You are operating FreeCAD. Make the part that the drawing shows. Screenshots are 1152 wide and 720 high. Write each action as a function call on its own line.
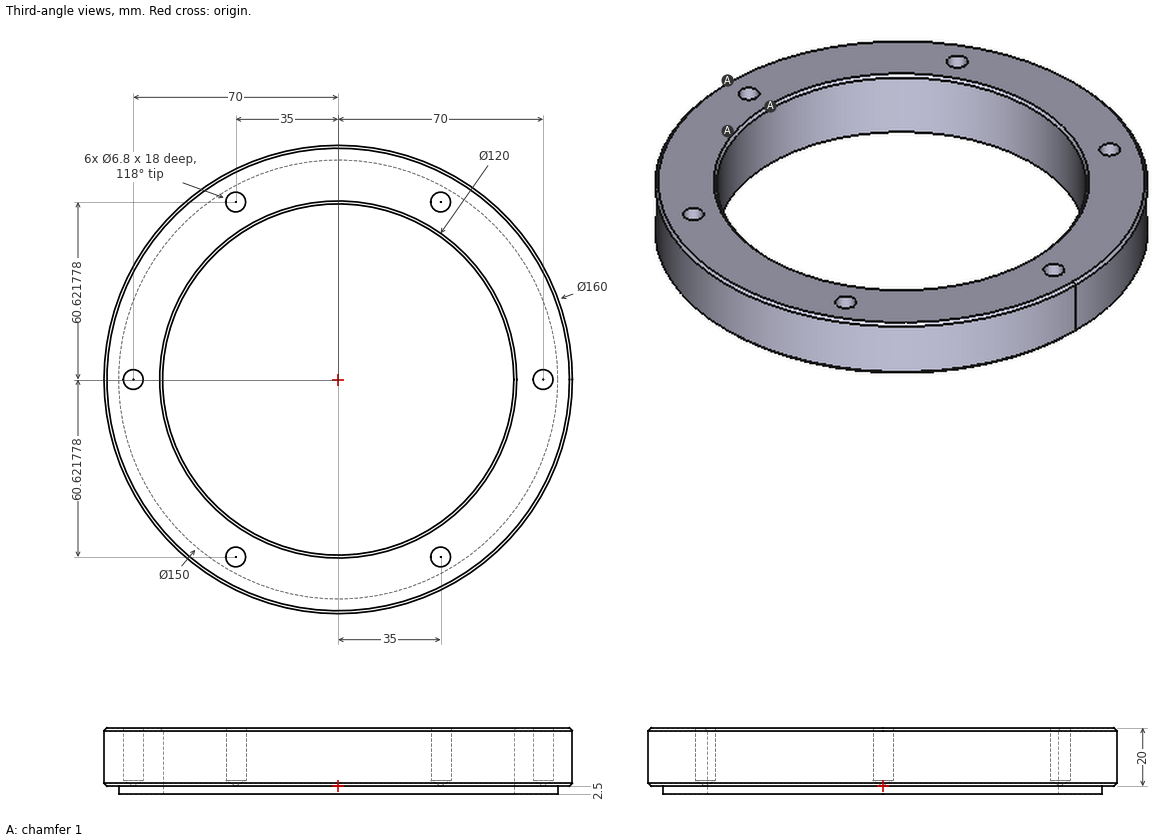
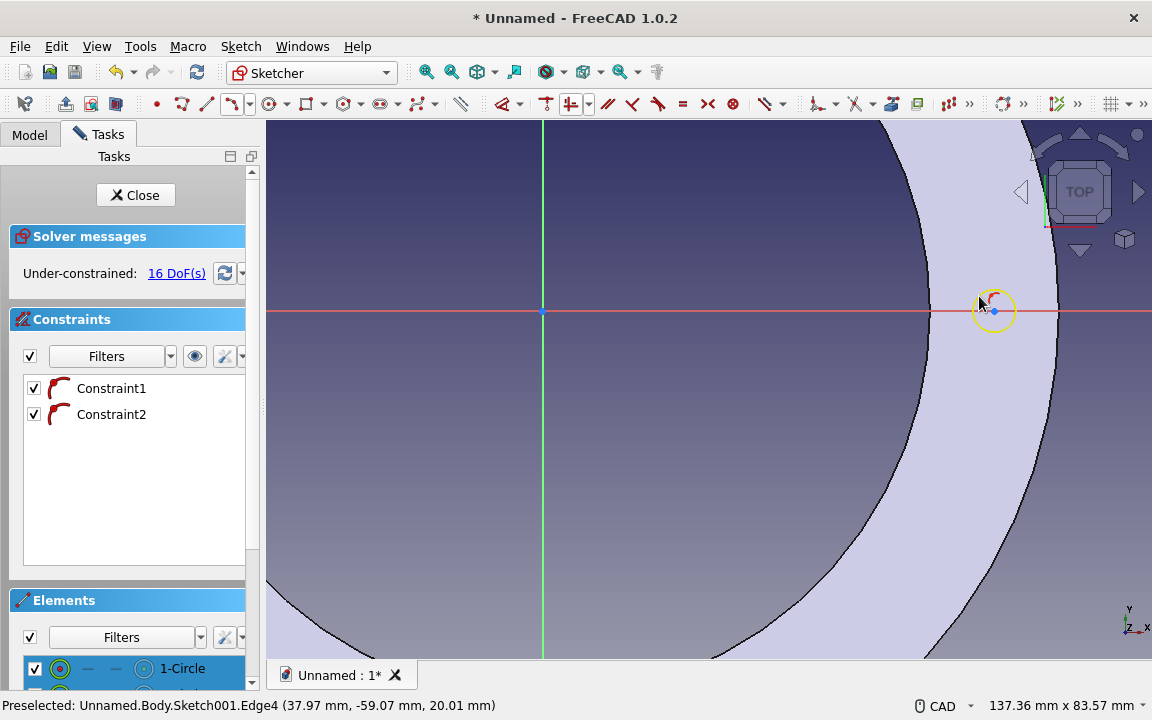
click(979, 296)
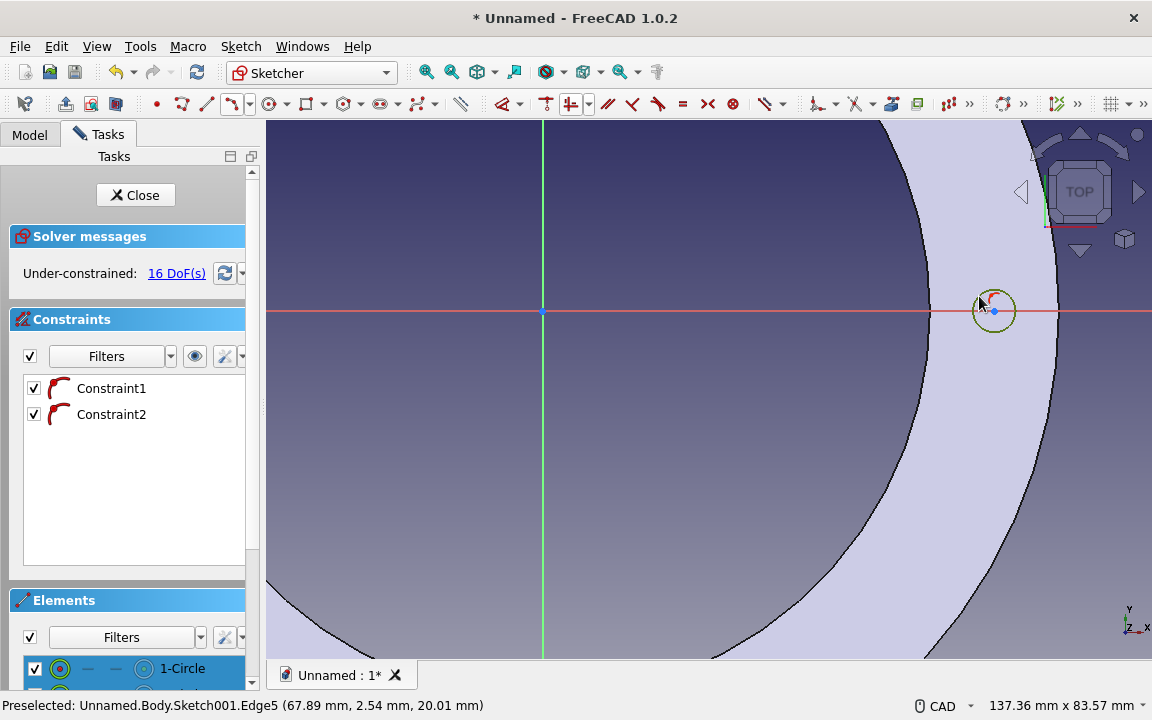
scroll(720, 454, down, 4)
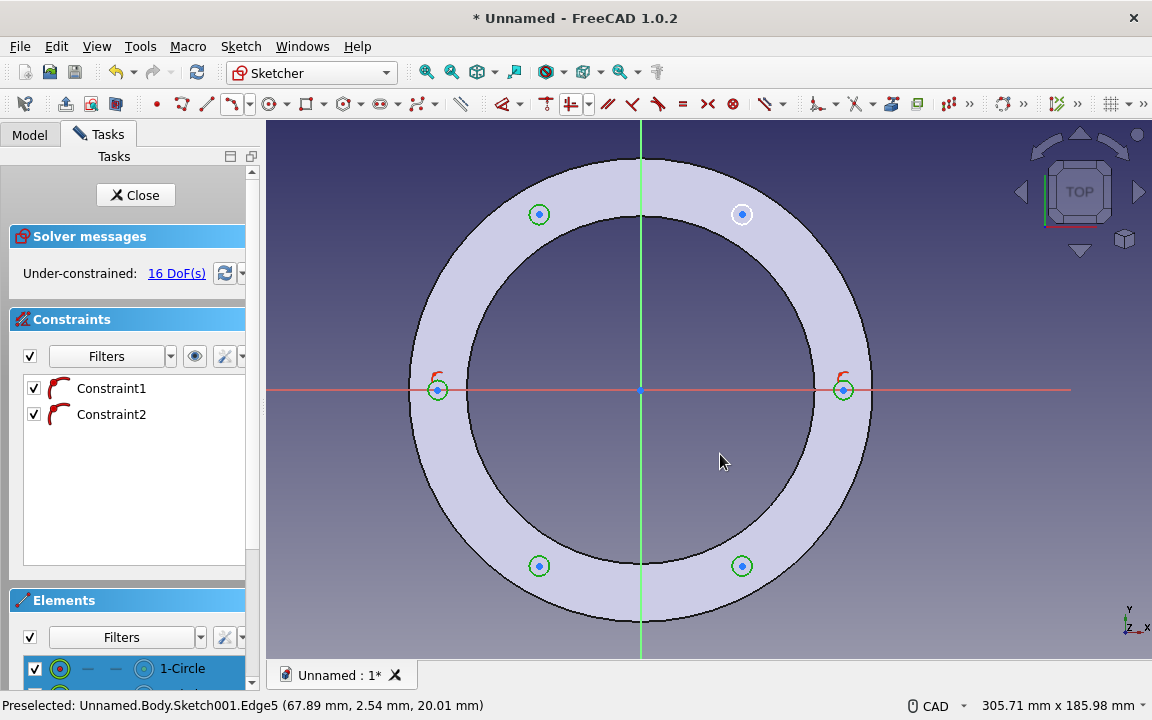
scroll(749, 208, up, 2)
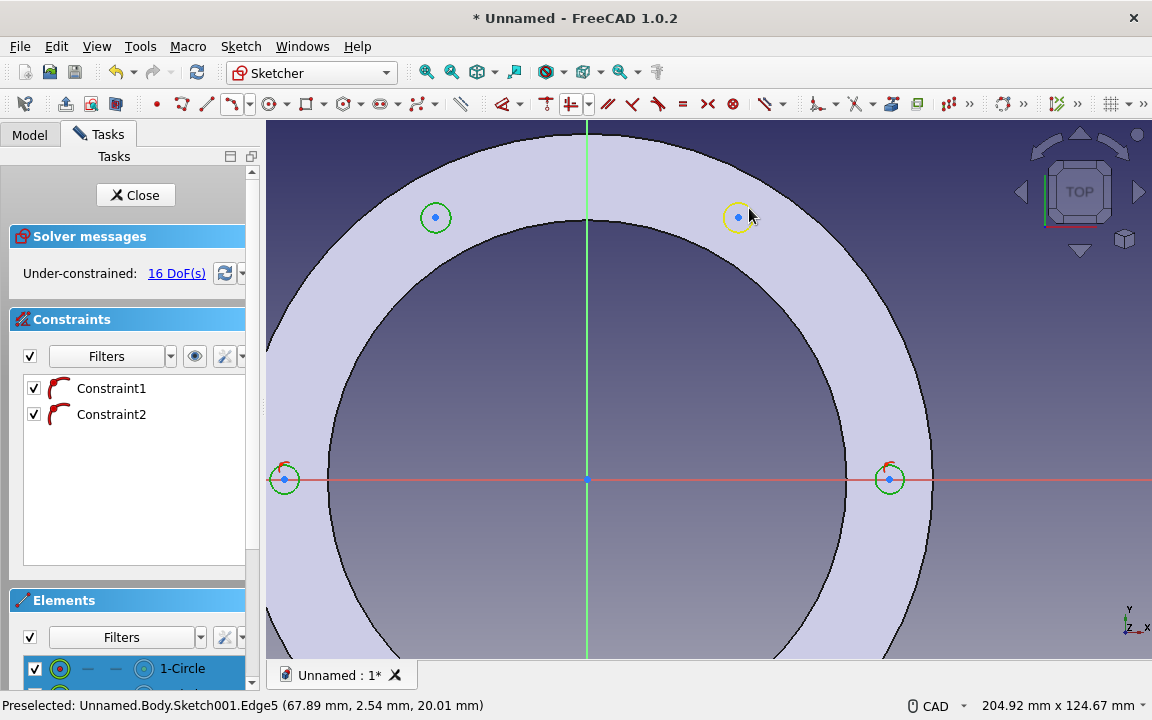
click(749, 207)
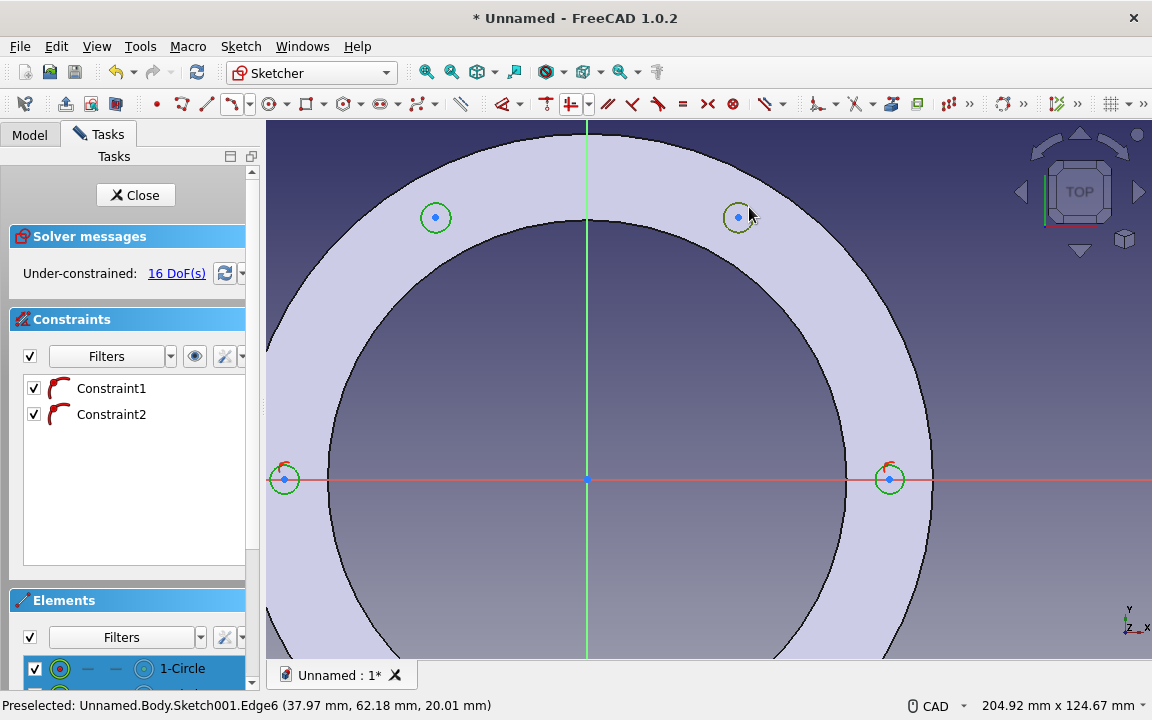
key(e)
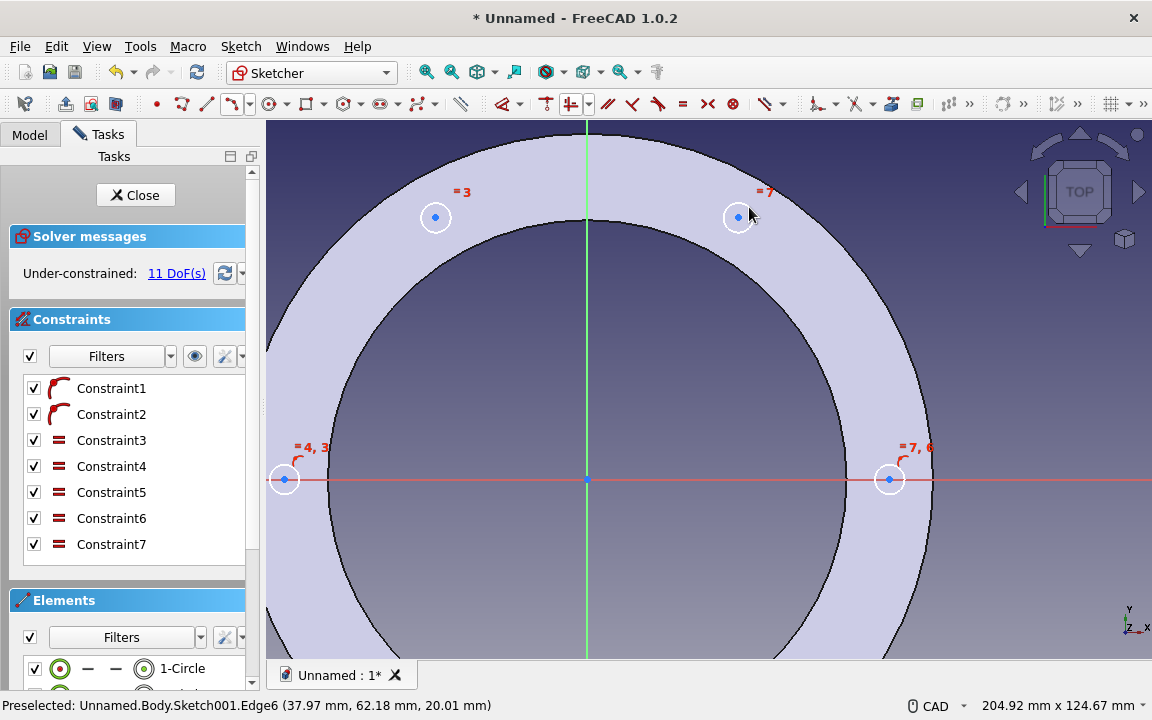
click(436, 218)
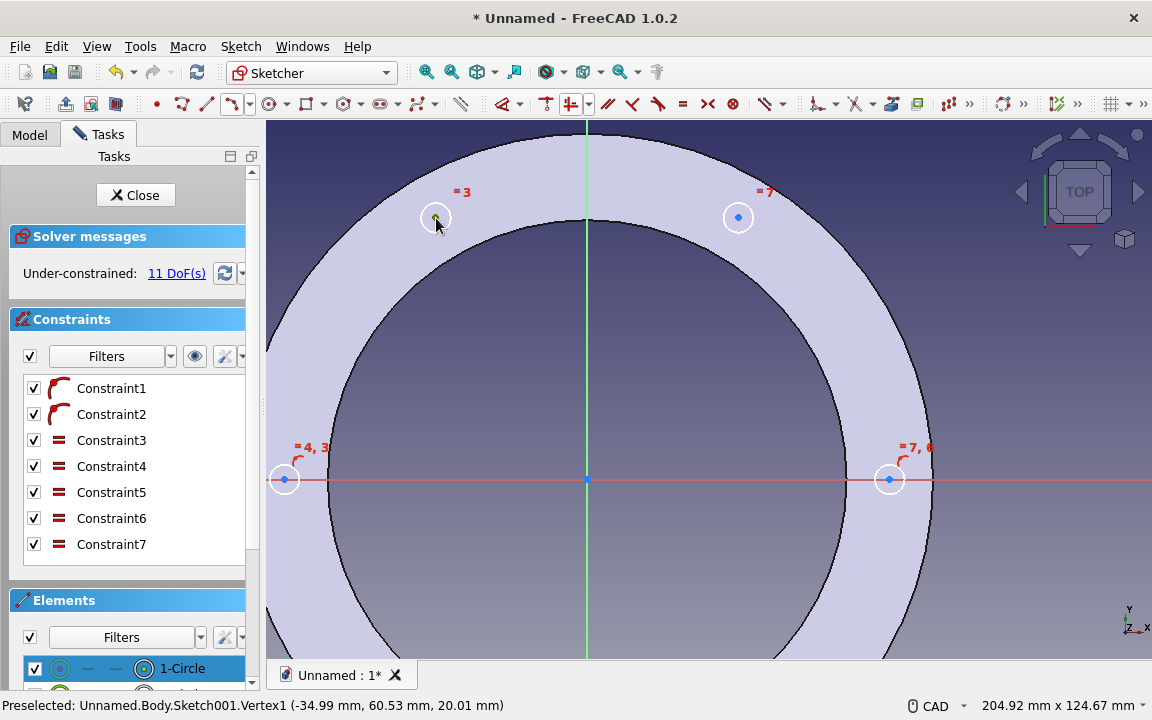
scroll(749, 206, down, 2)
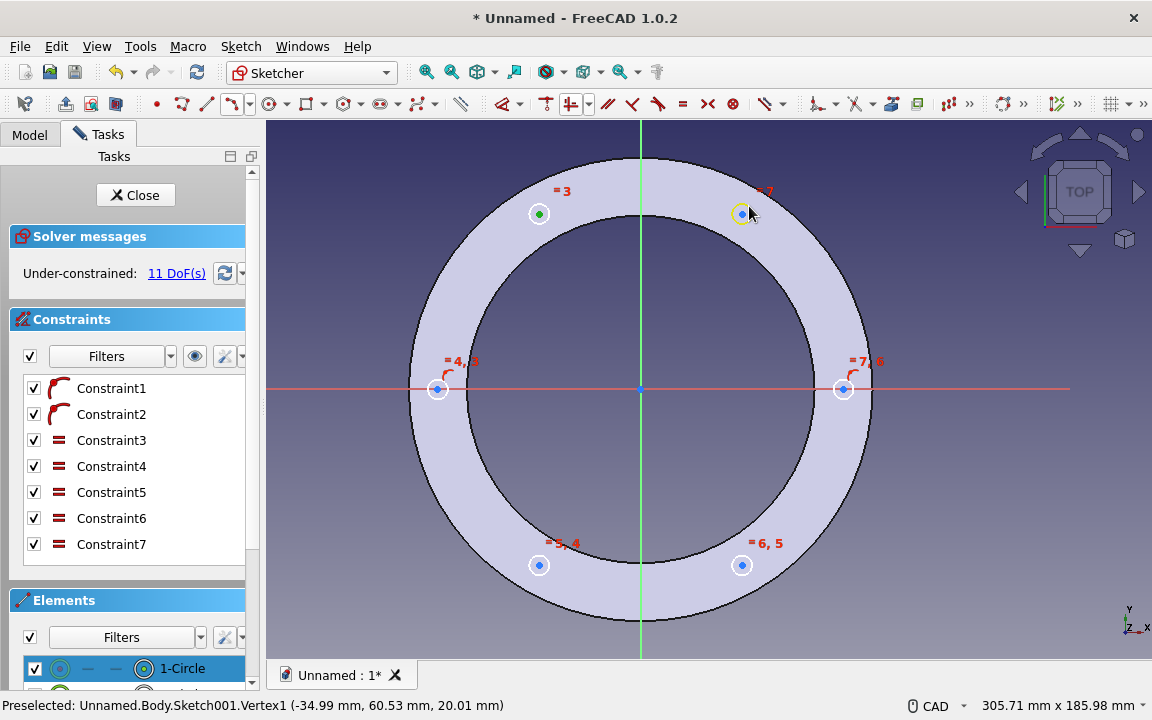
click(539, 565)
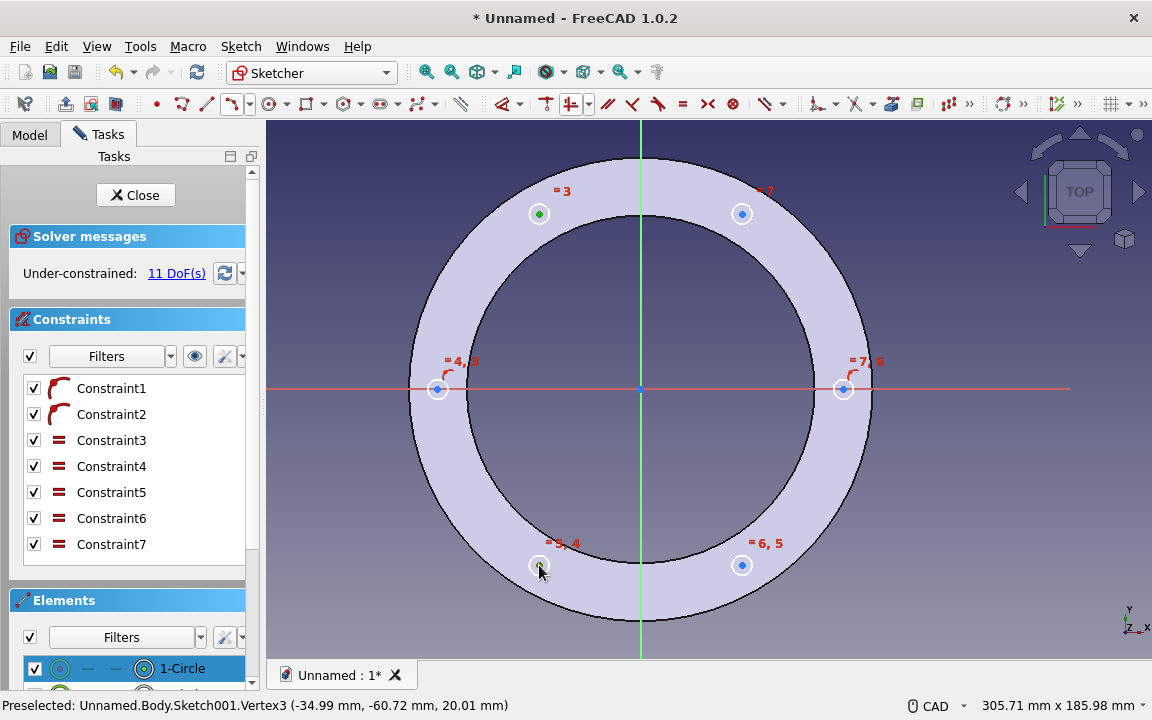
click(588, 104)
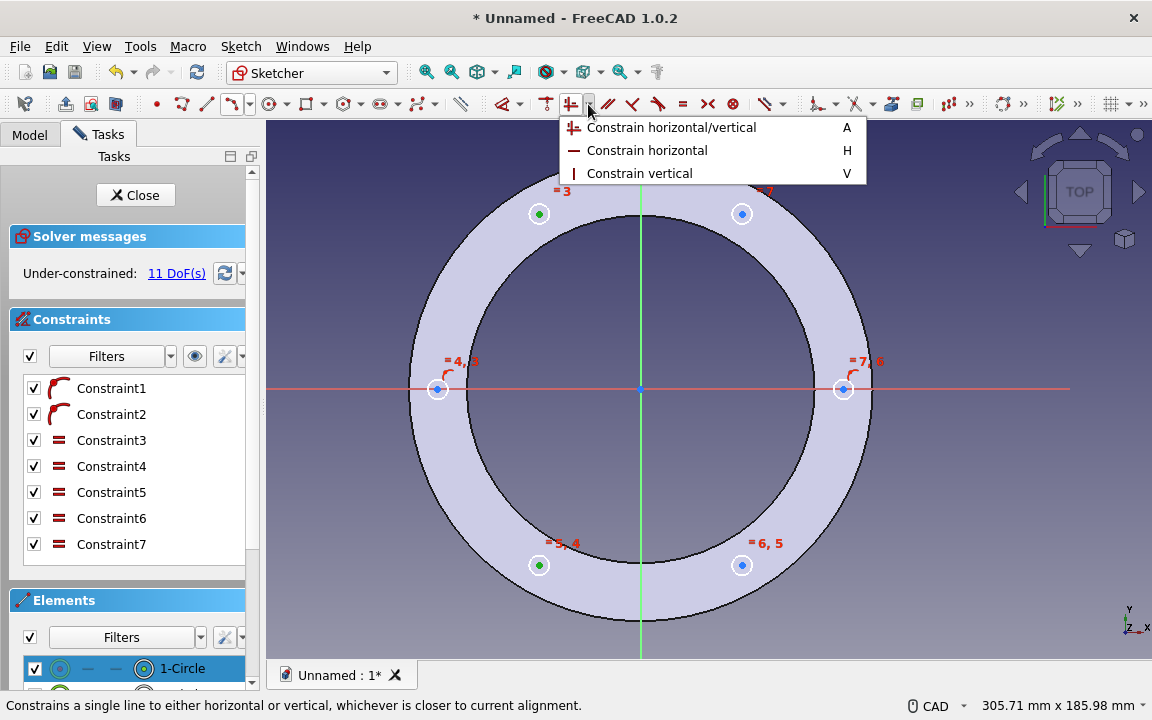
click(713, 174)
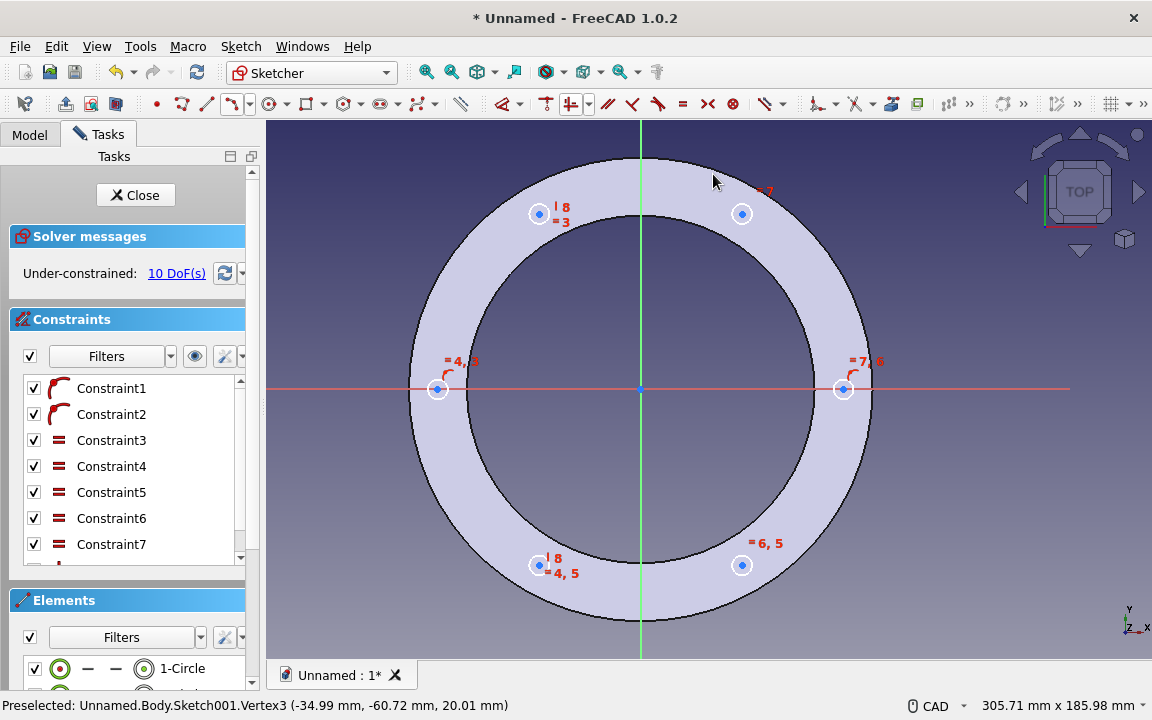
click(539, 565)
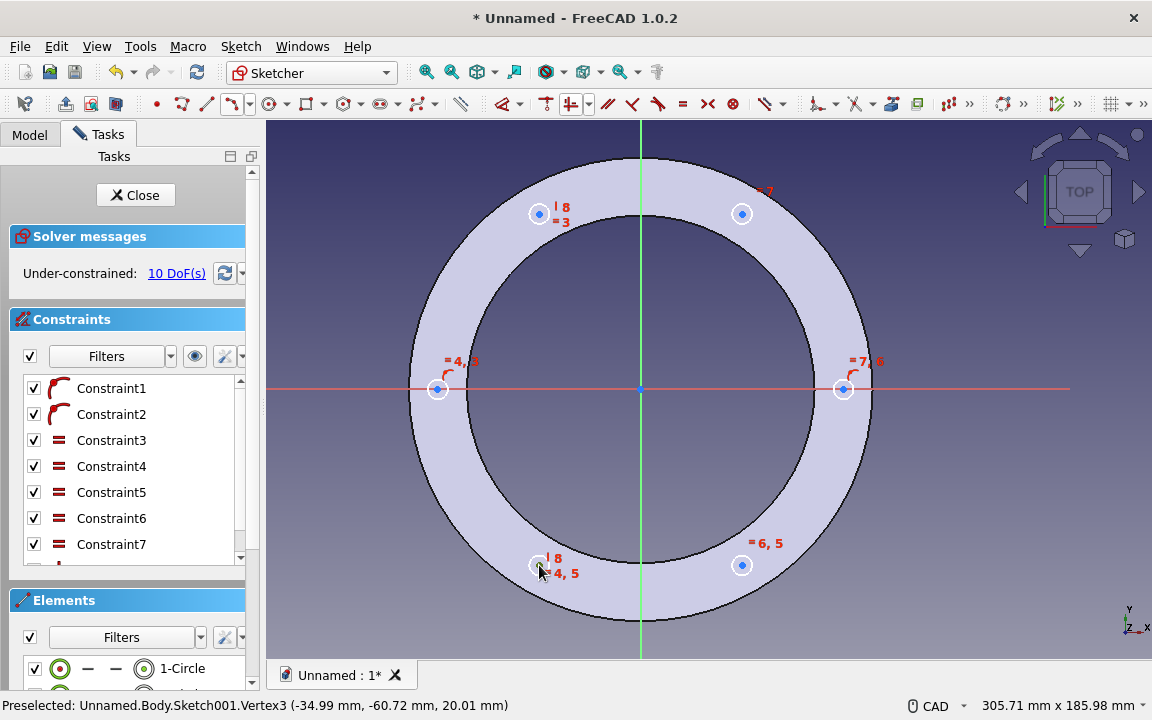
click(742, 565)